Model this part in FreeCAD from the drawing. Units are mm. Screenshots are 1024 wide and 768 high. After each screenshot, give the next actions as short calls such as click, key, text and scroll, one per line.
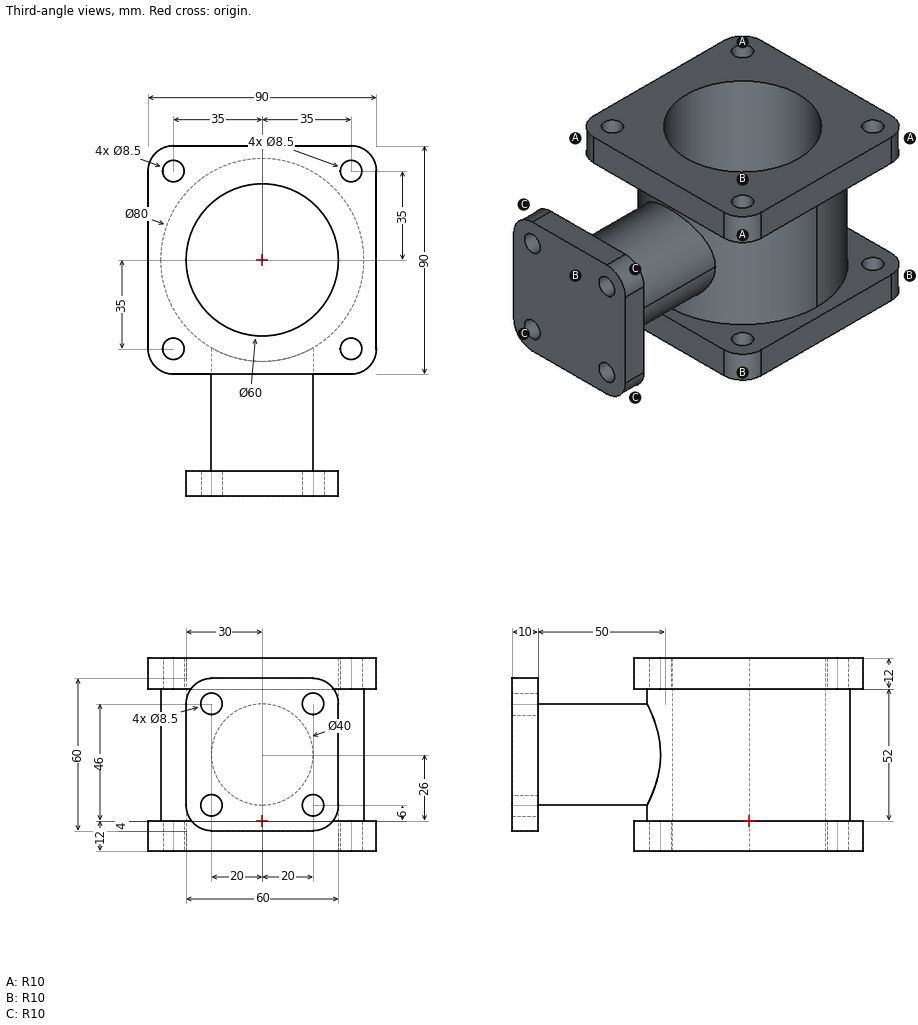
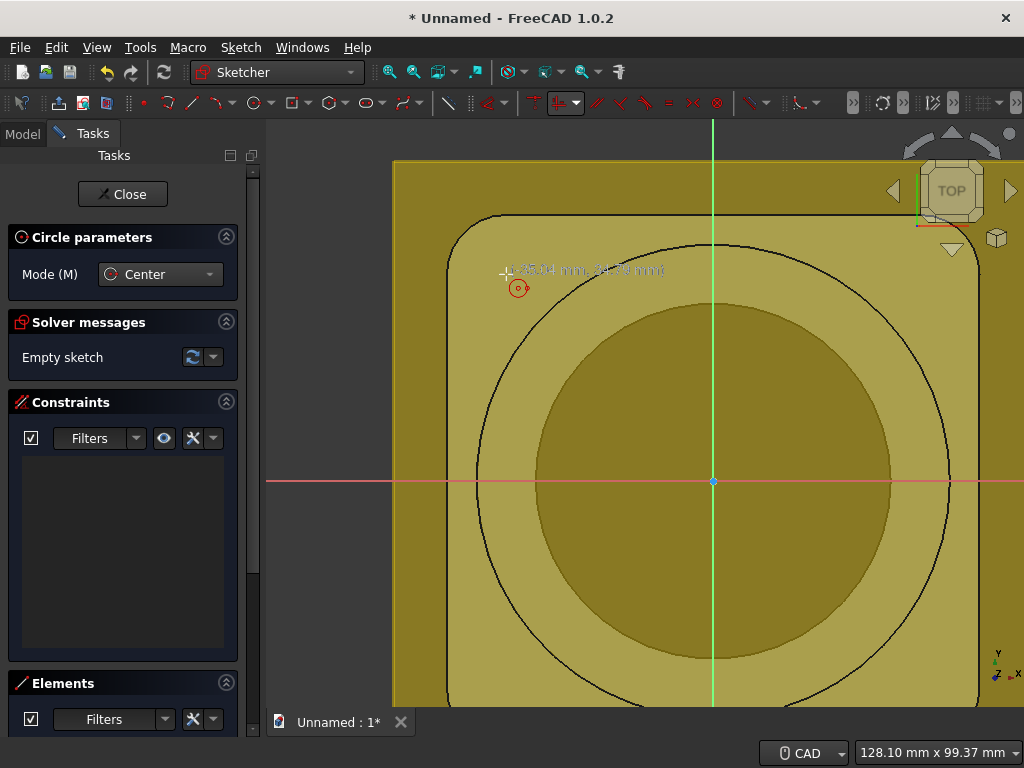
click(506, 274)
click(524, 256)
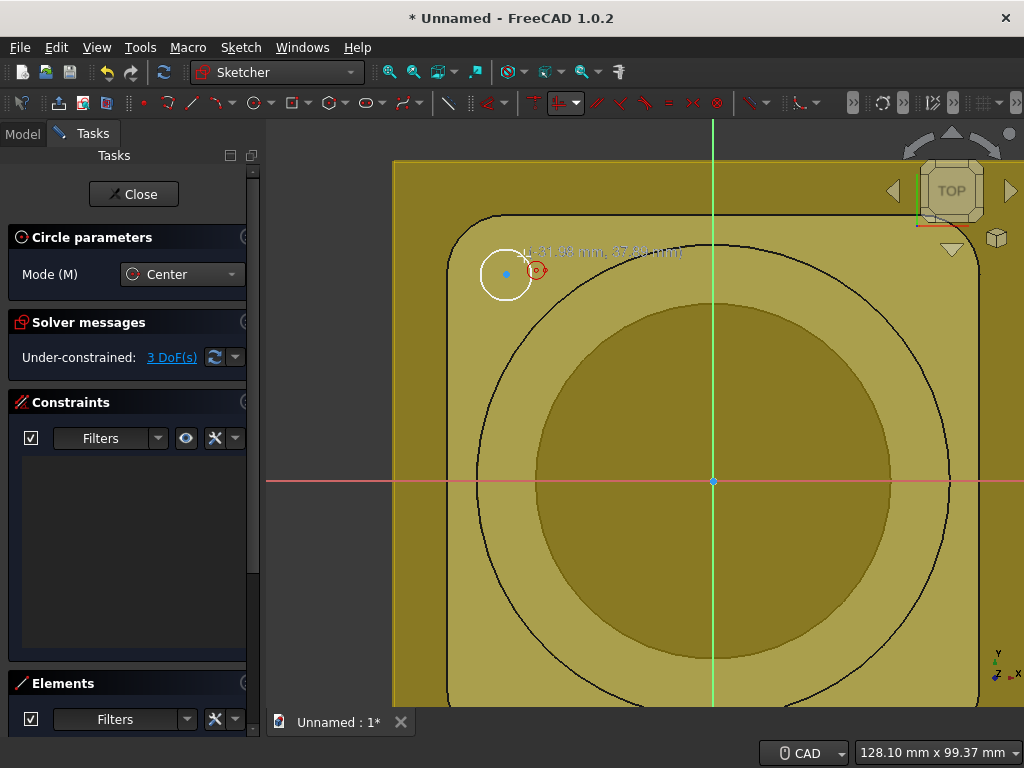
scroll(294, 147, down, 1)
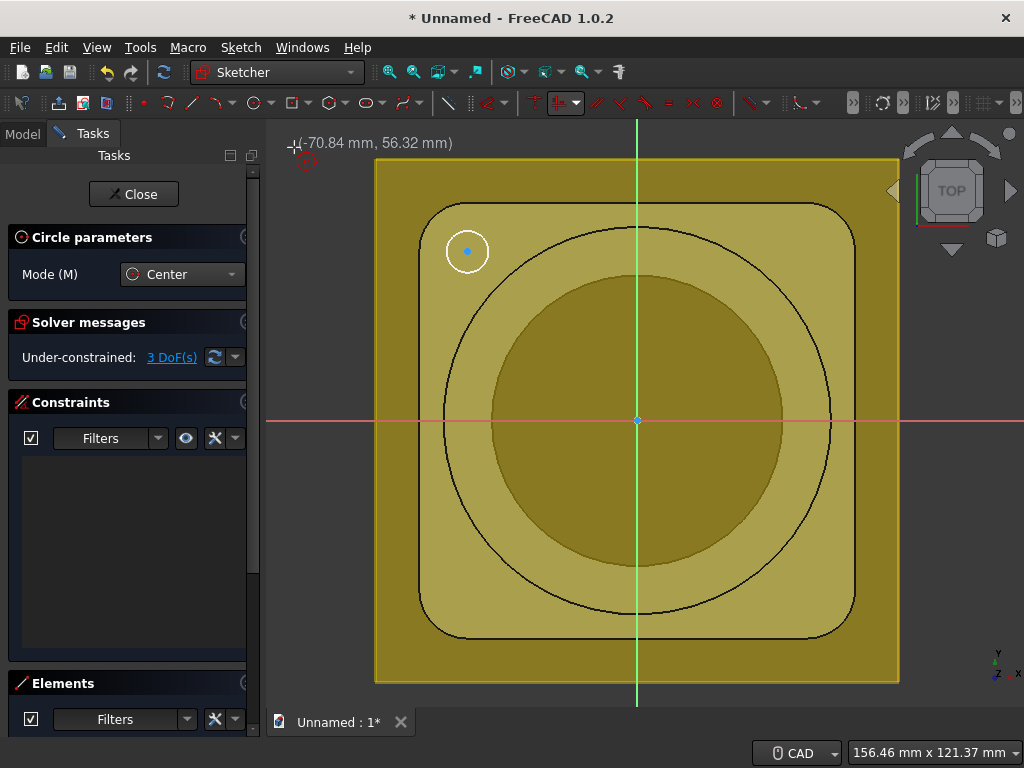
click(807, 251)
click(821, 237)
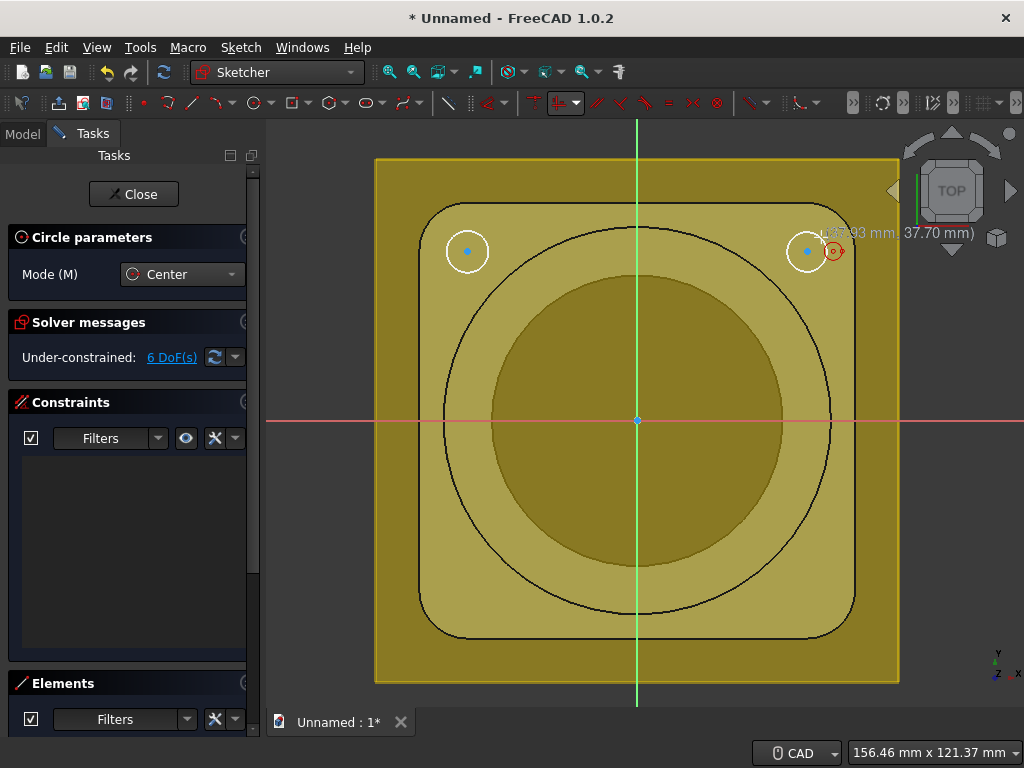
click(807, 590)
click(821, 576)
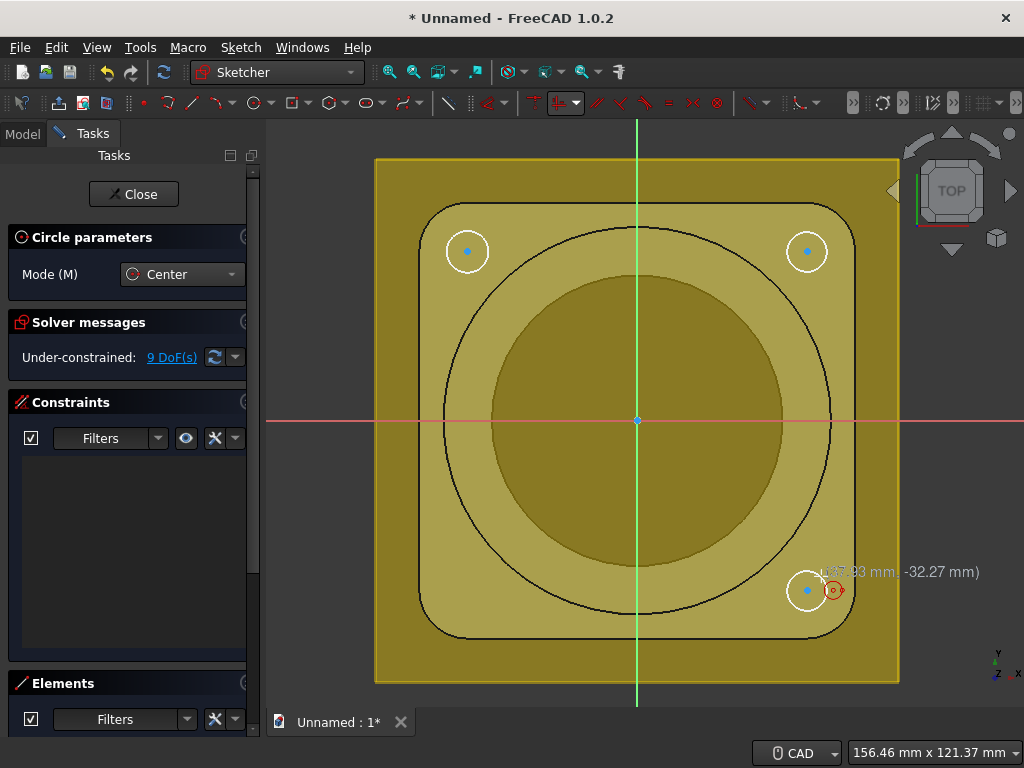
click(468, 590)
click(482, 576)
key(Escape)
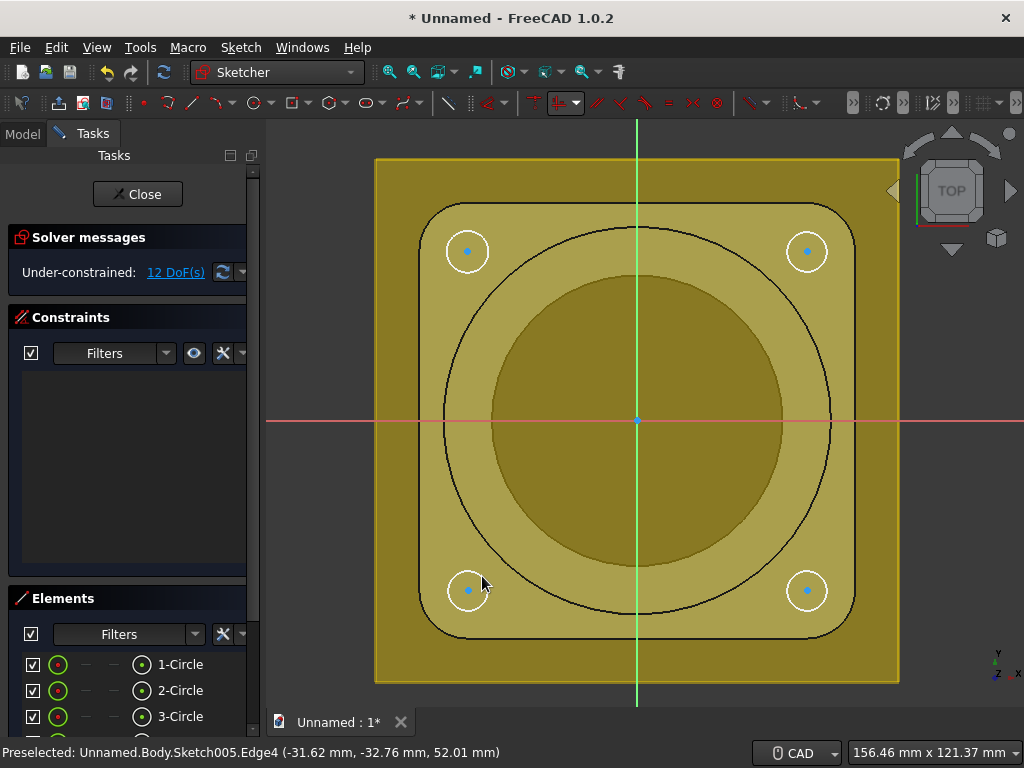
click(482, 237)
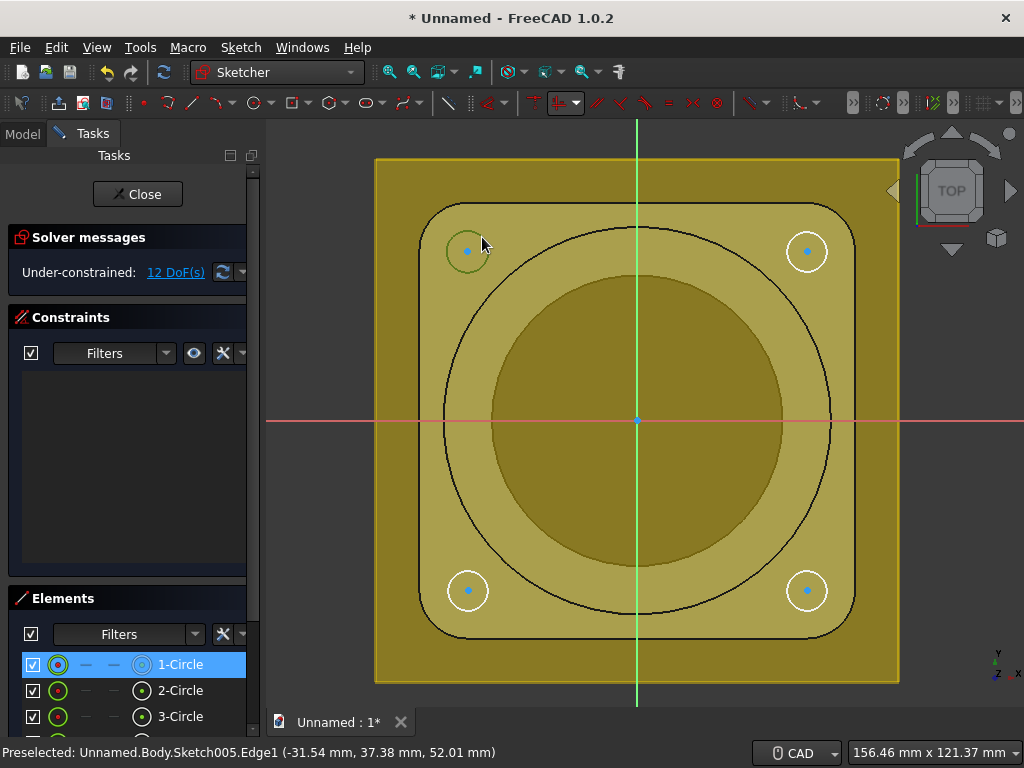
click(821, 238)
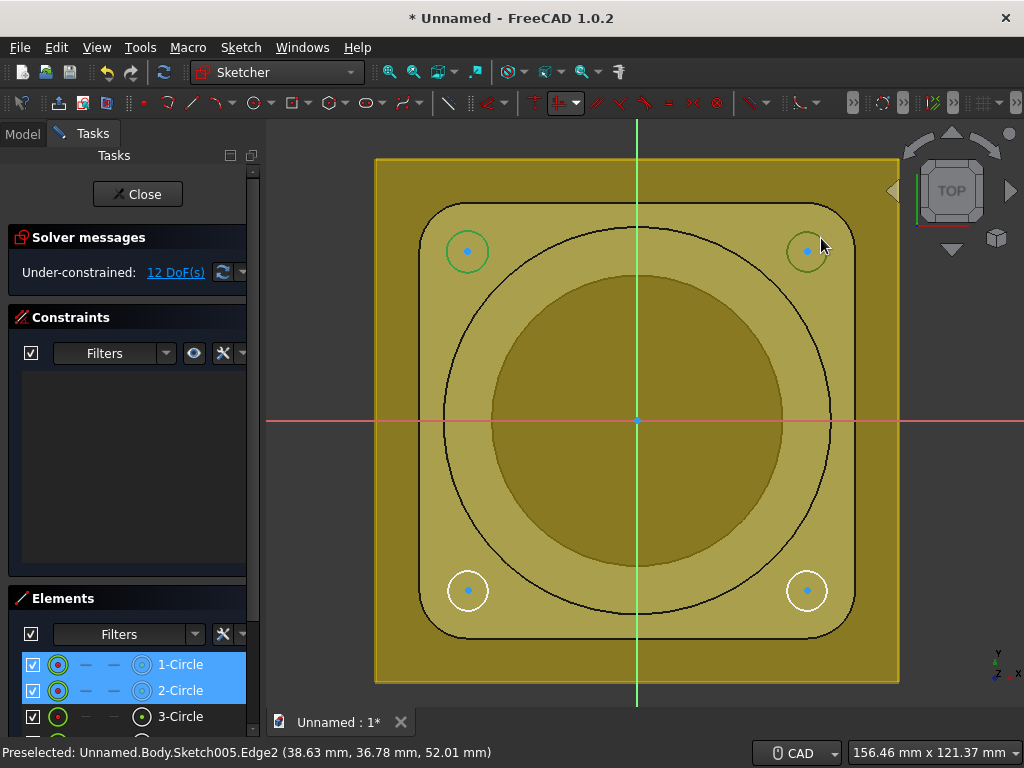
click(821, 577)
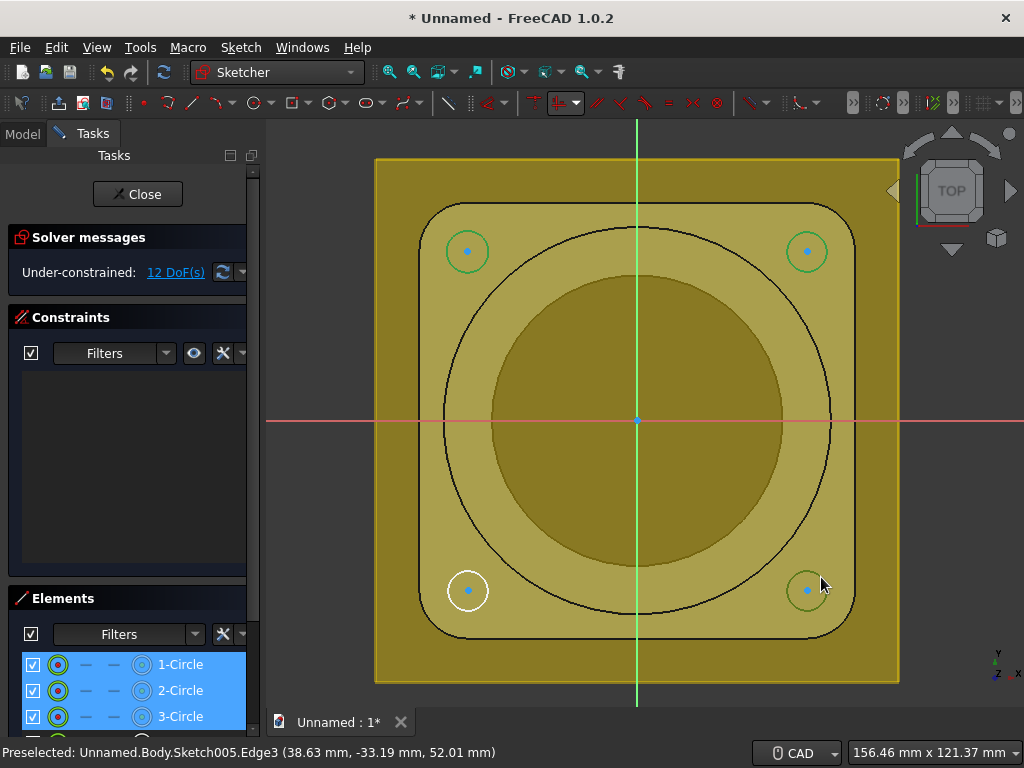
click(482, 577)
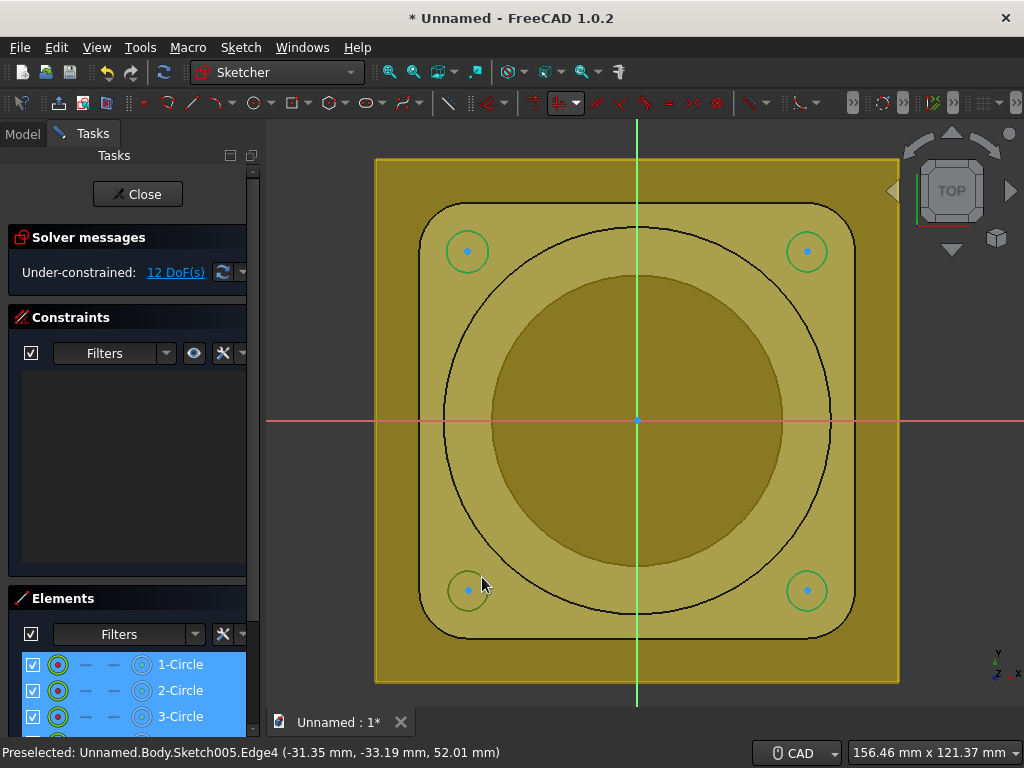
click(670, 104)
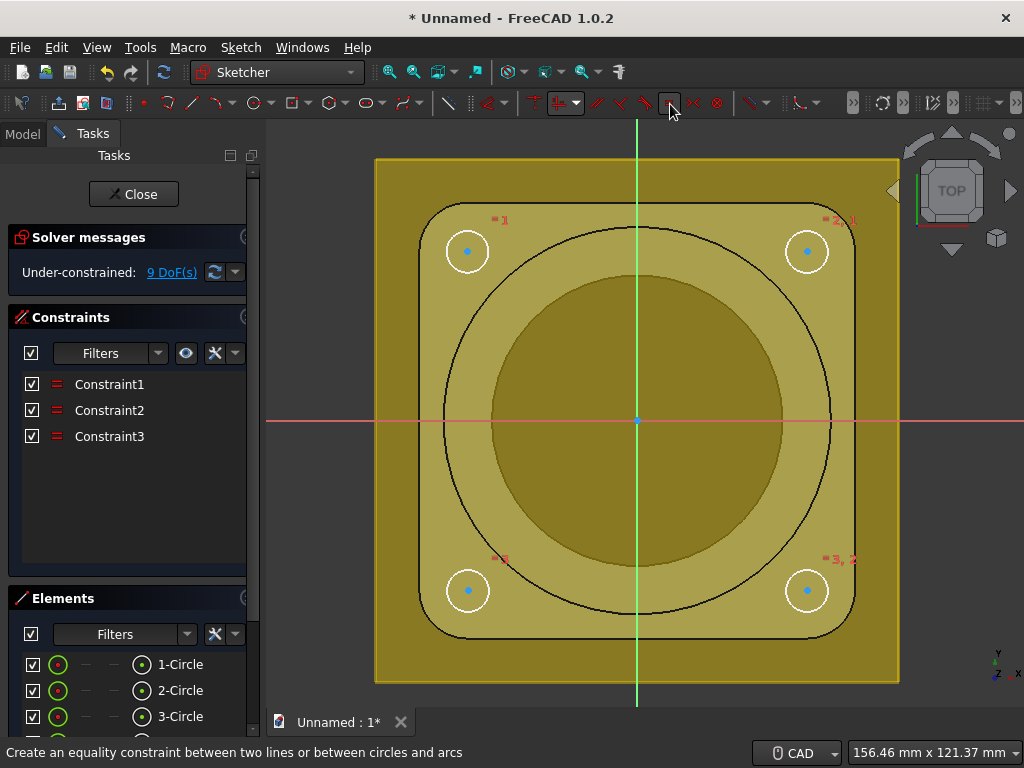
click(468, 252)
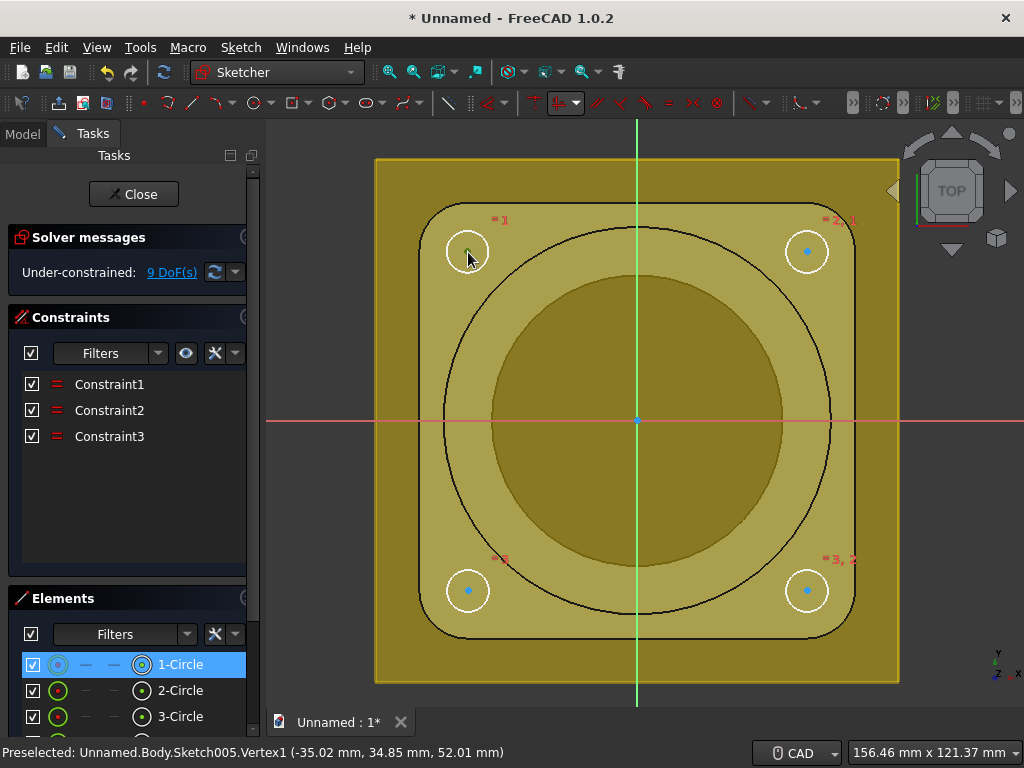
click(807, 252)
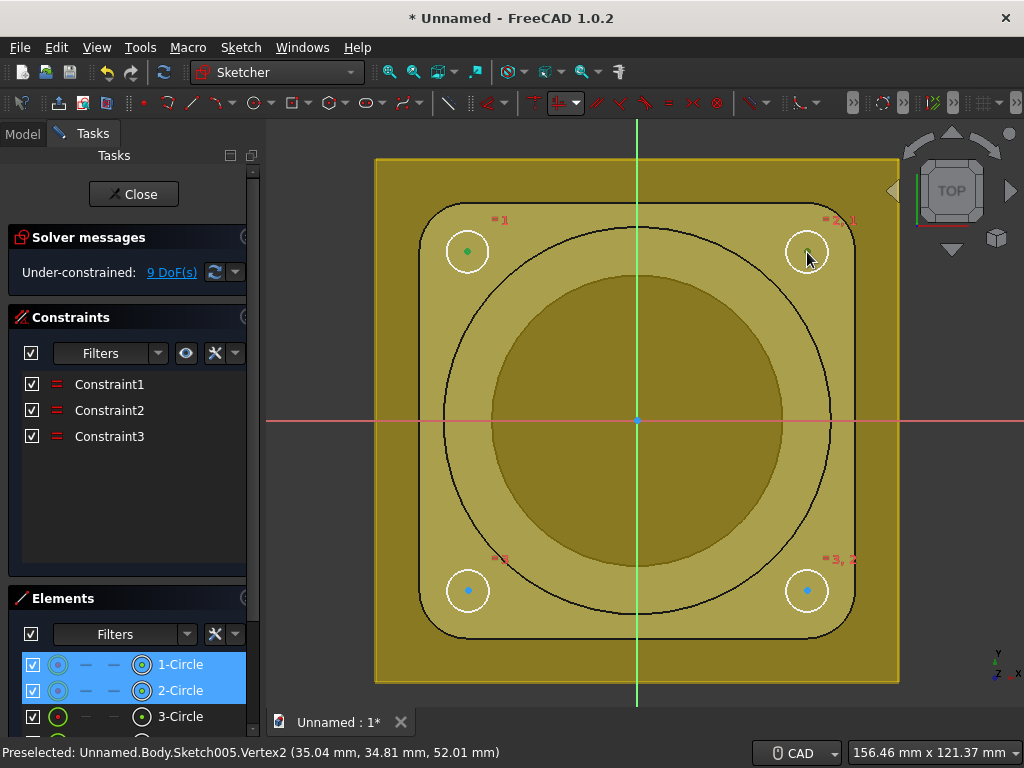
click(578, 104)